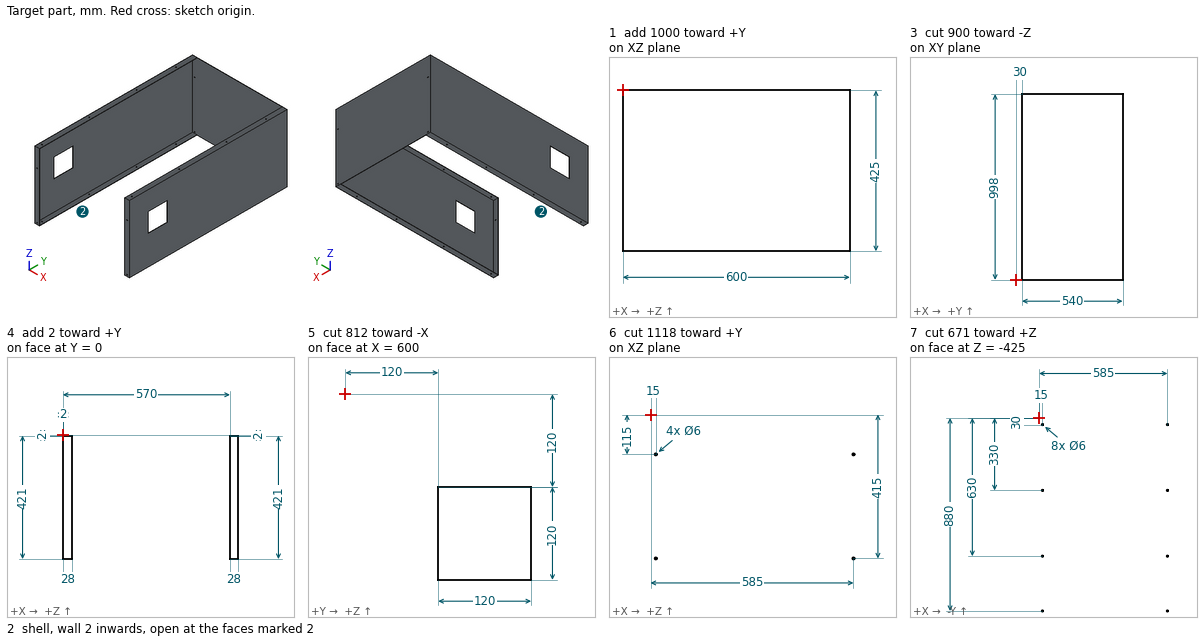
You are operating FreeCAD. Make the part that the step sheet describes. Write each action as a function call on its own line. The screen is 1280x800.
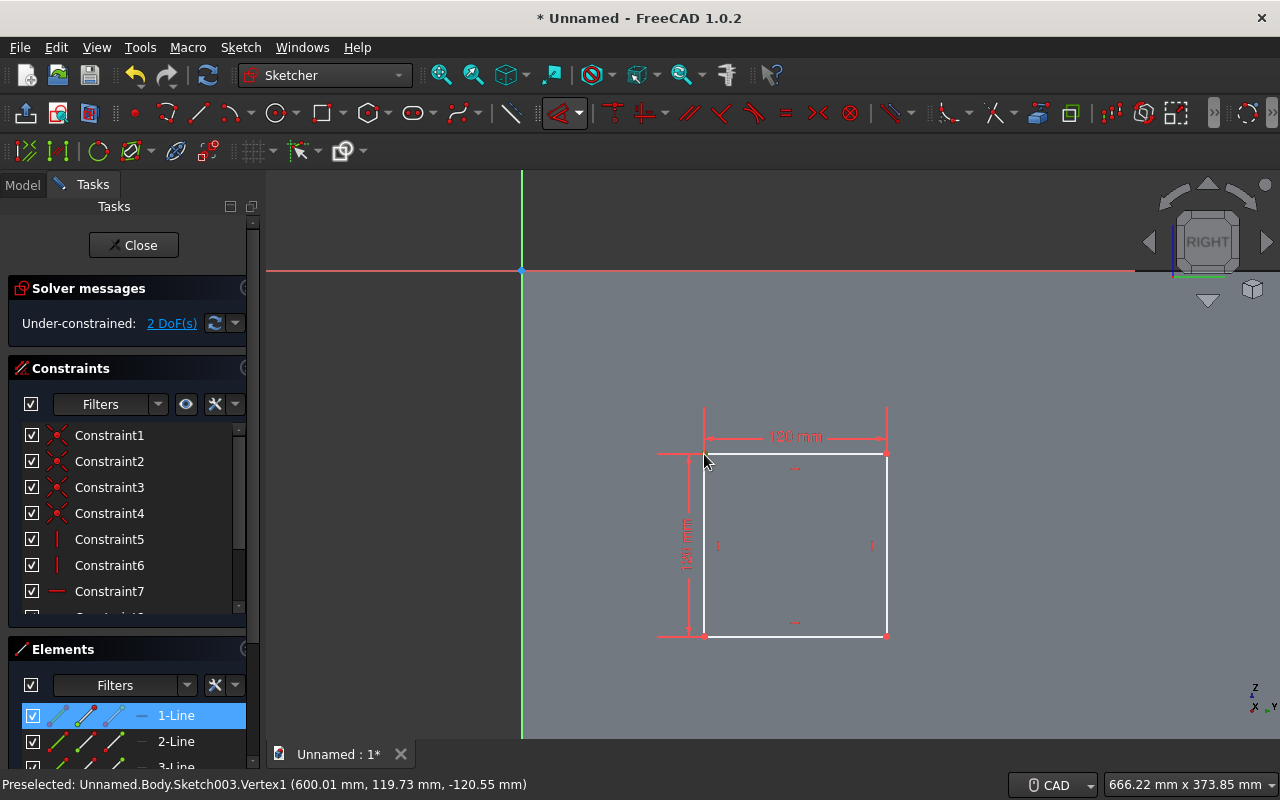
click(582, 114)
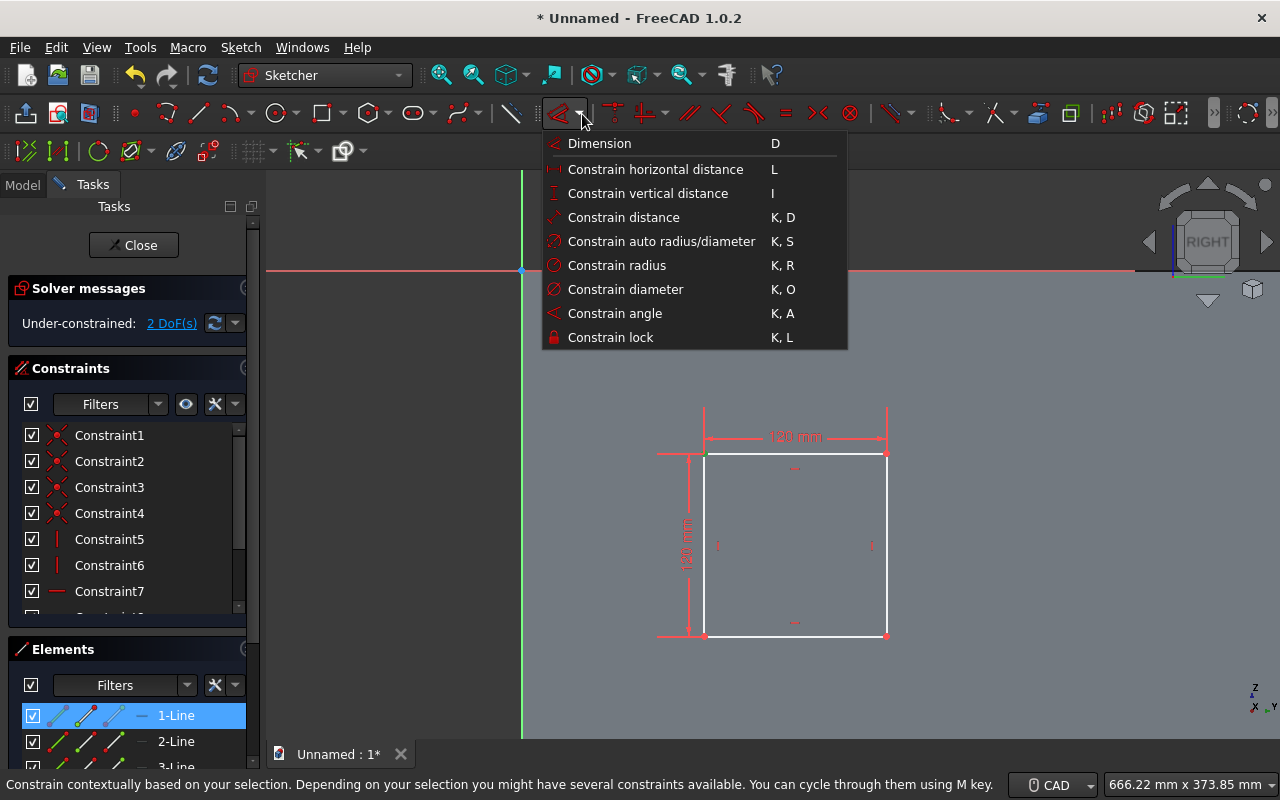
click(695, 169)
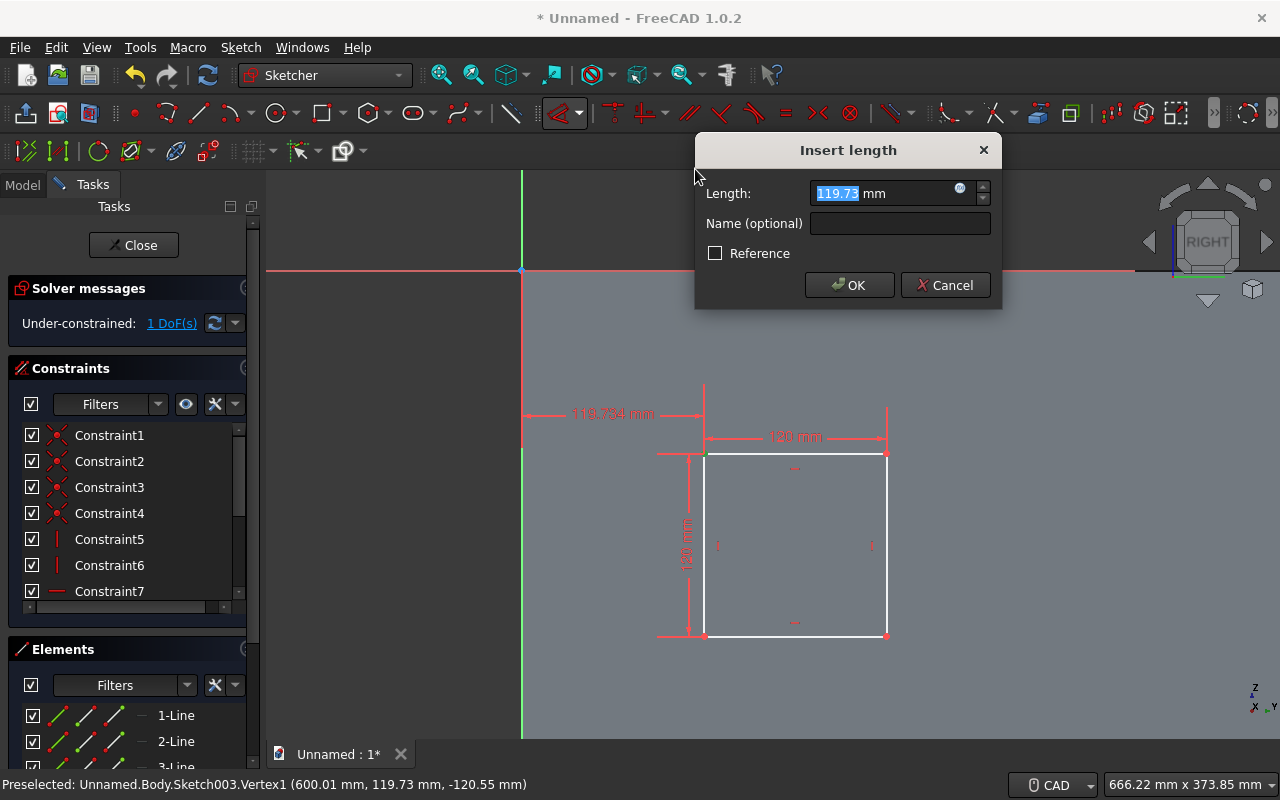
text(120)
key(Return)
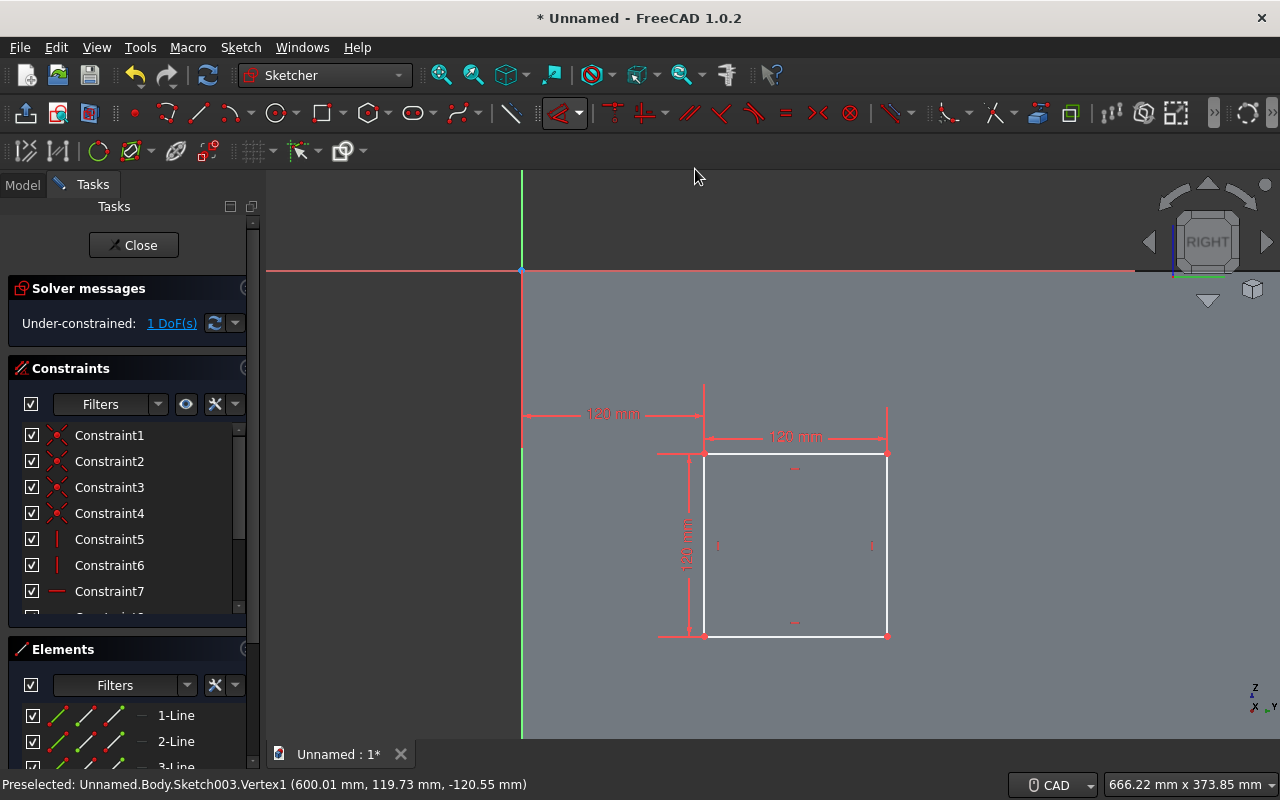
click(704, 454)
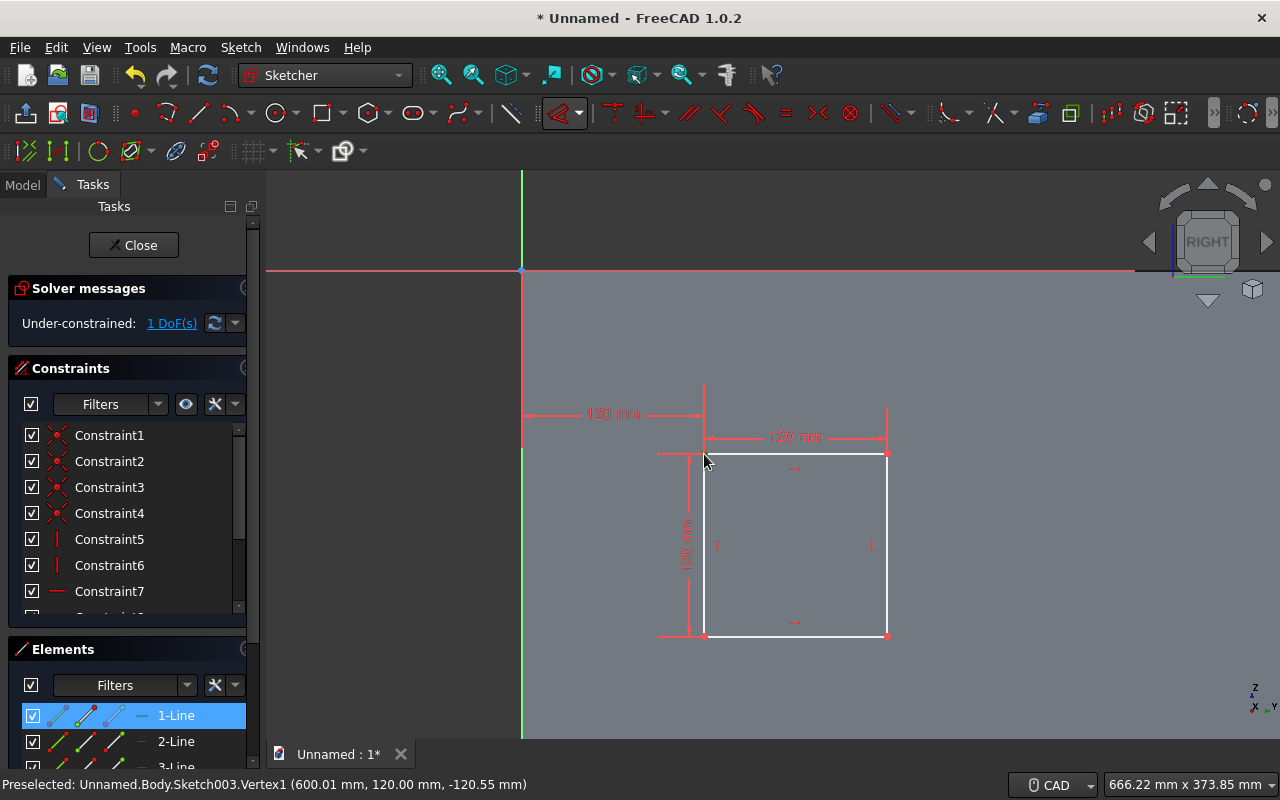
click(582, 114)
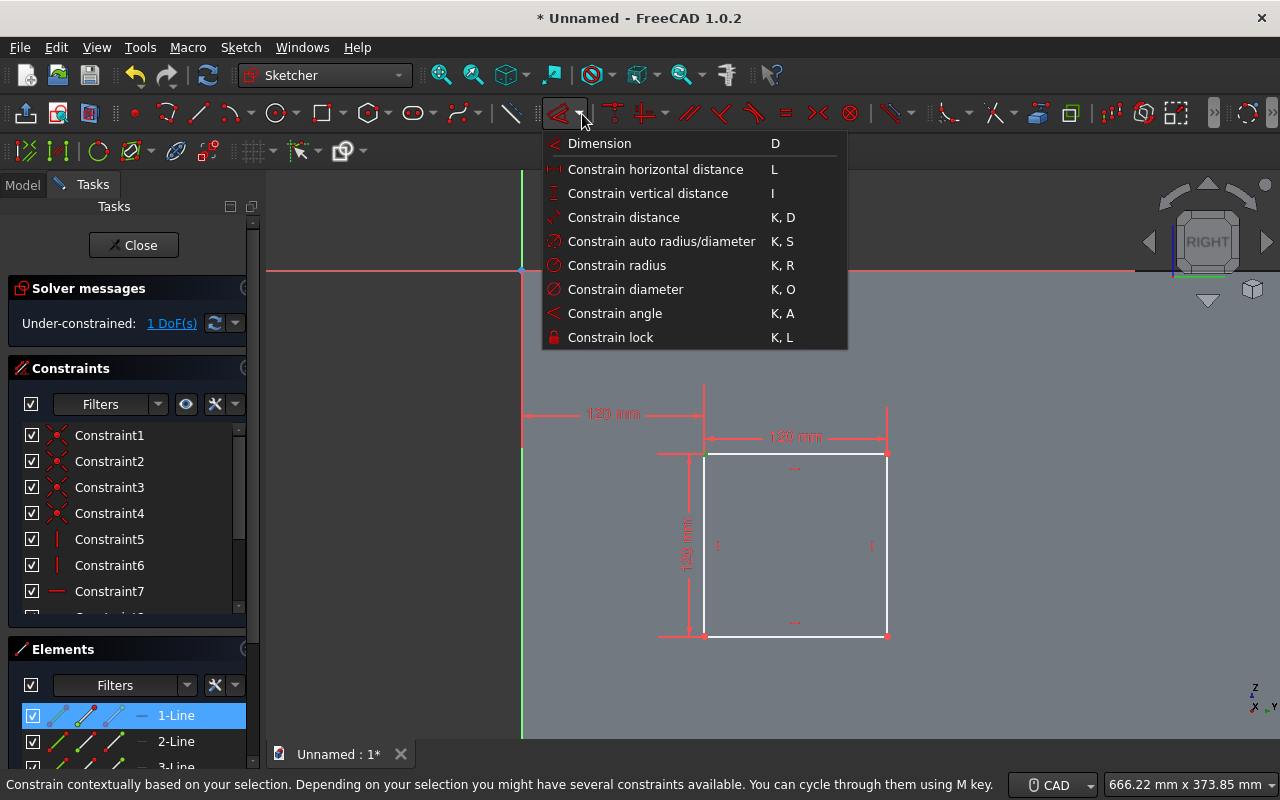
click(695, 193)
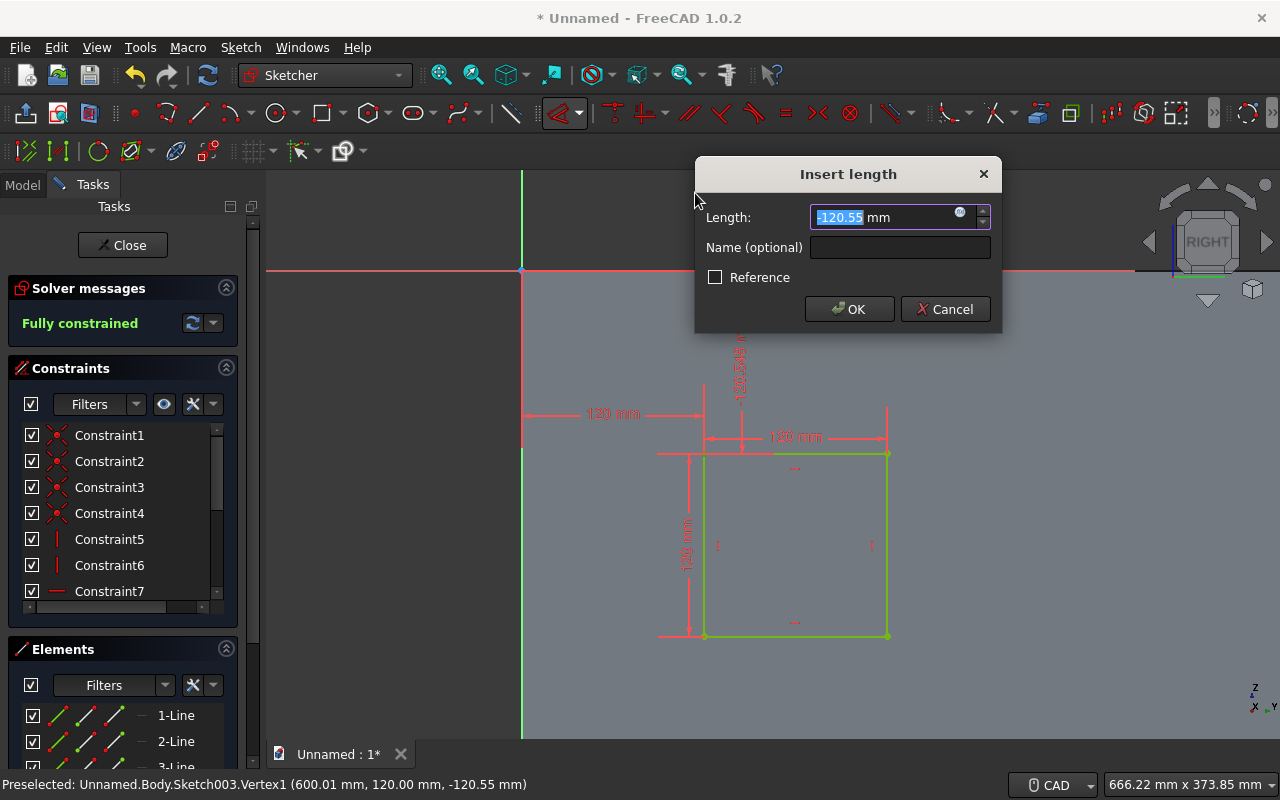
text(-120)
key(Return)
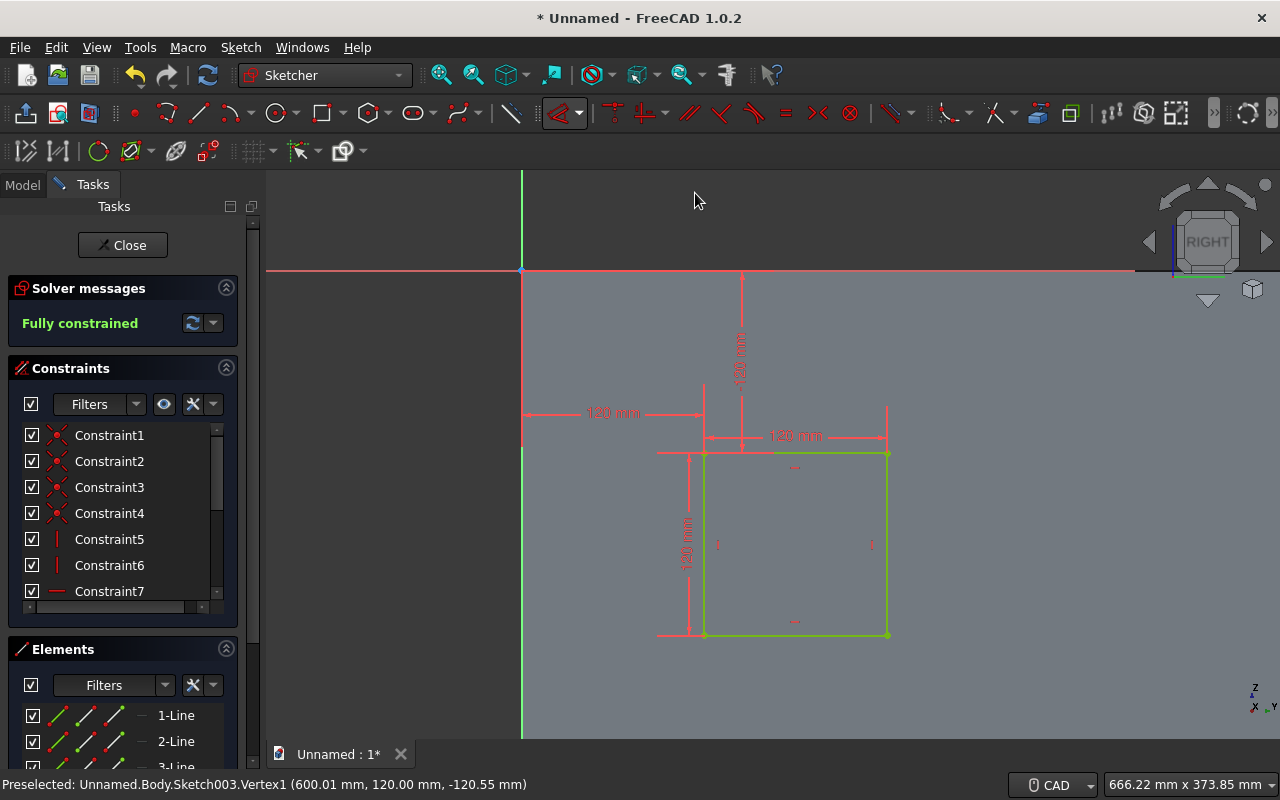
click(123, 245)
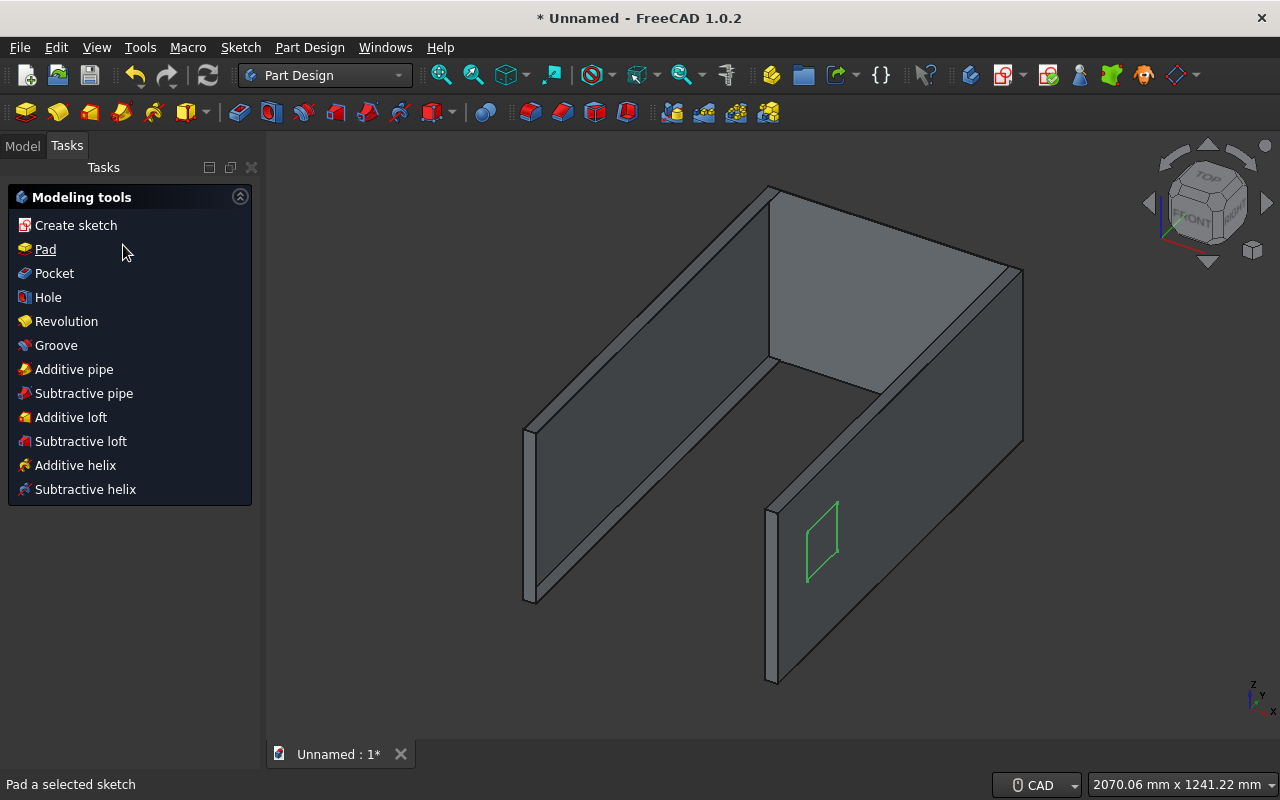
click(240, 112)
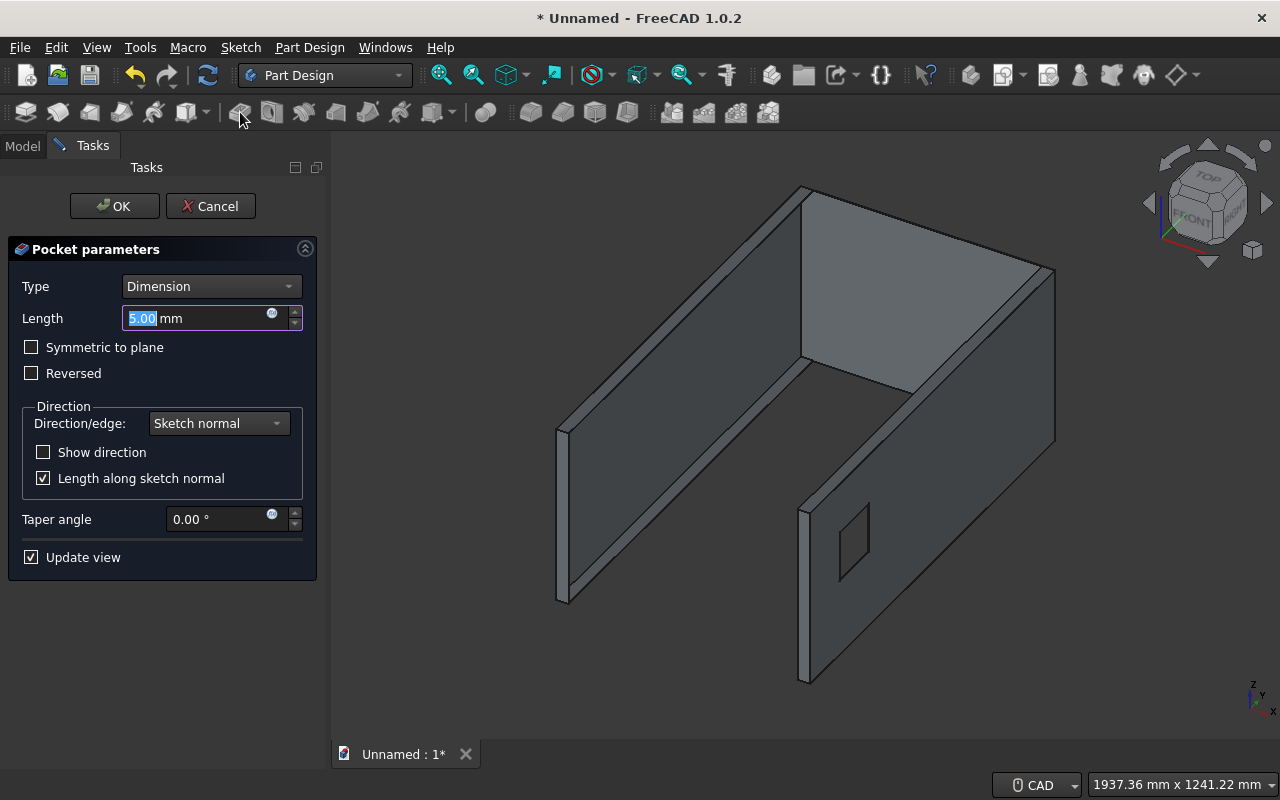
text(812)
key(Tab)